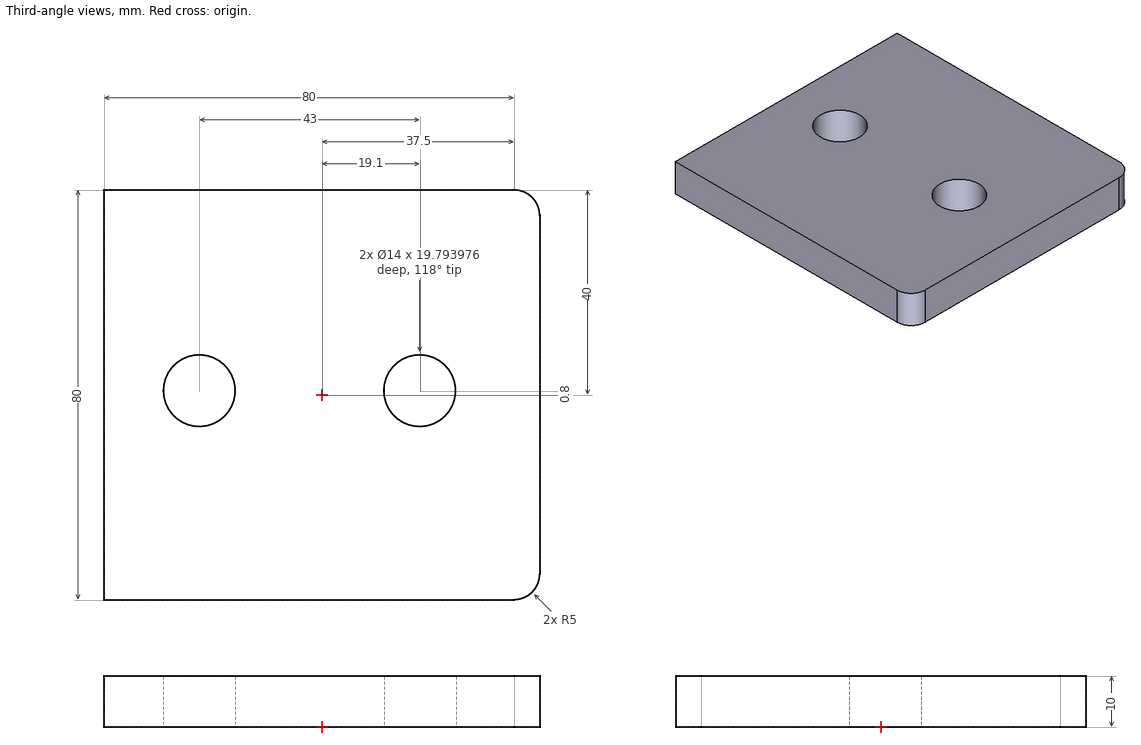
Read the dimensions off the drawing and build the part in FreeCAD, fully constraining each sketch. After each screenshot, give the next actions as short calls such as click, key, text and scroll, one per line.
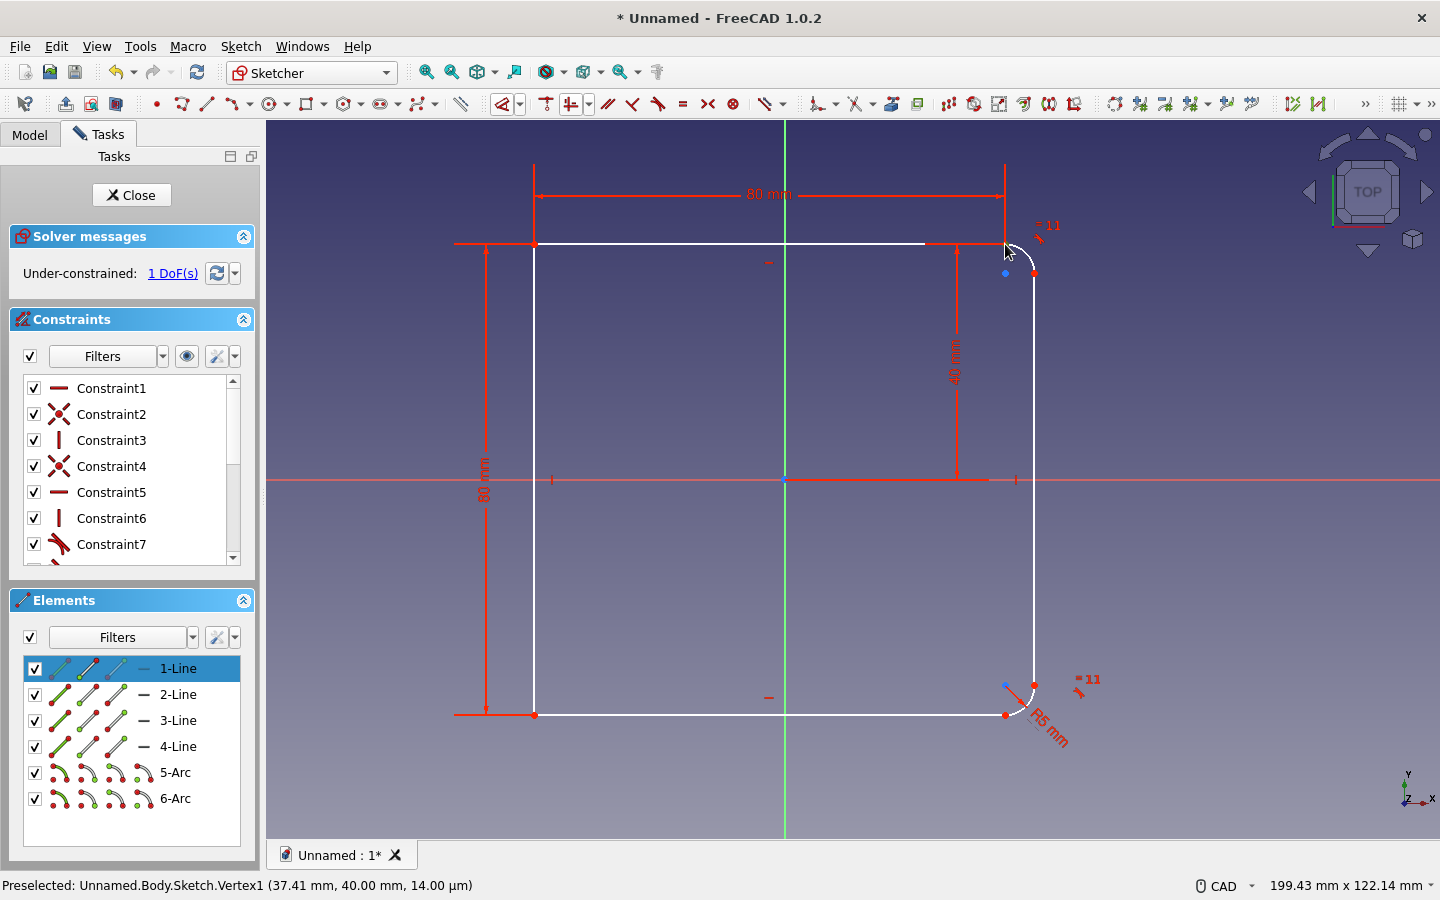
click(520, 104)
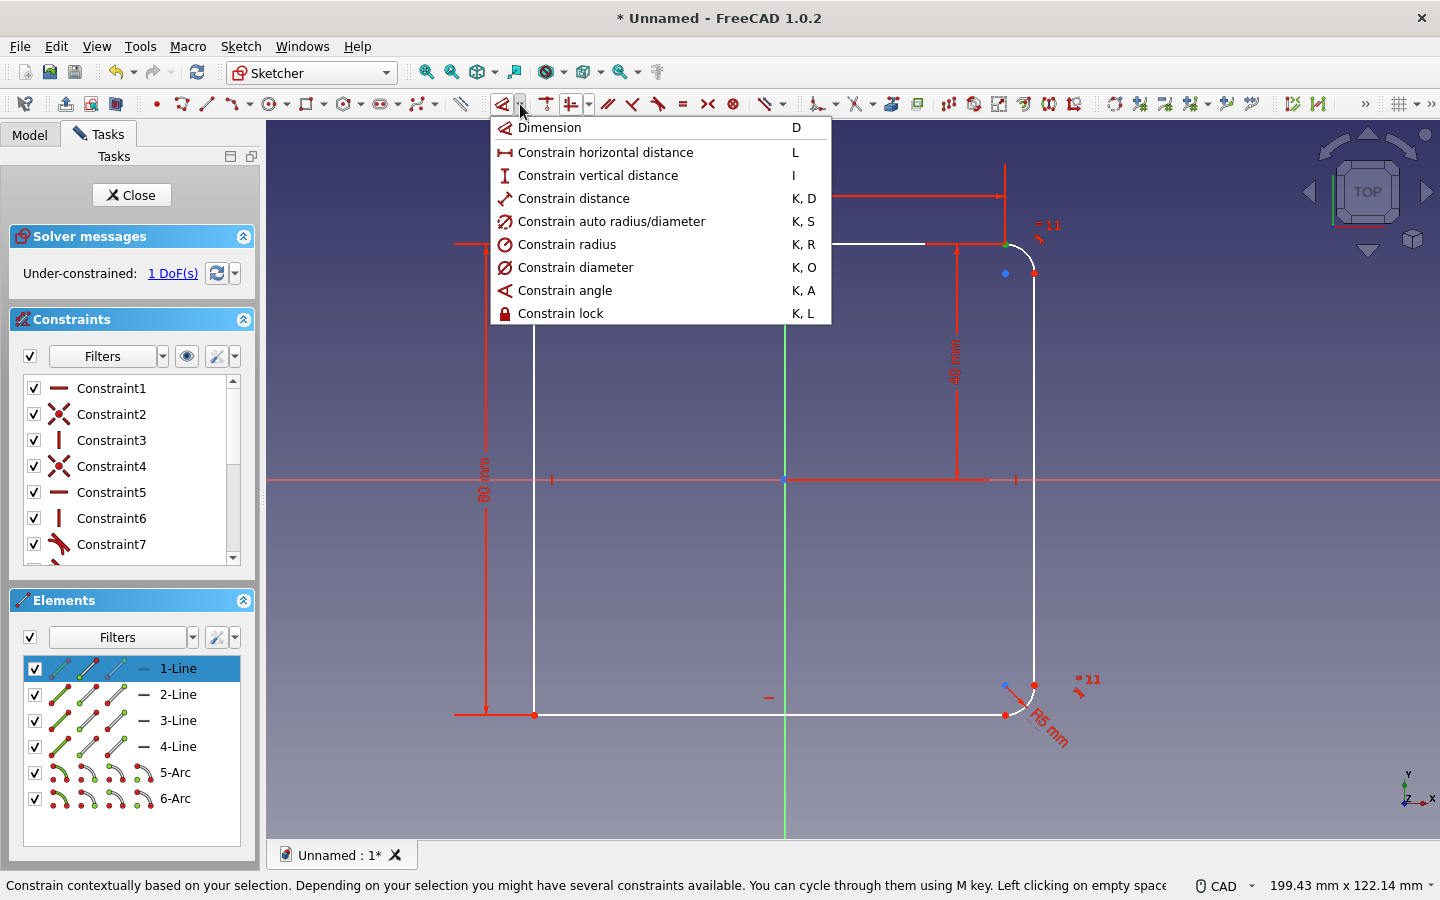
click(661, 152)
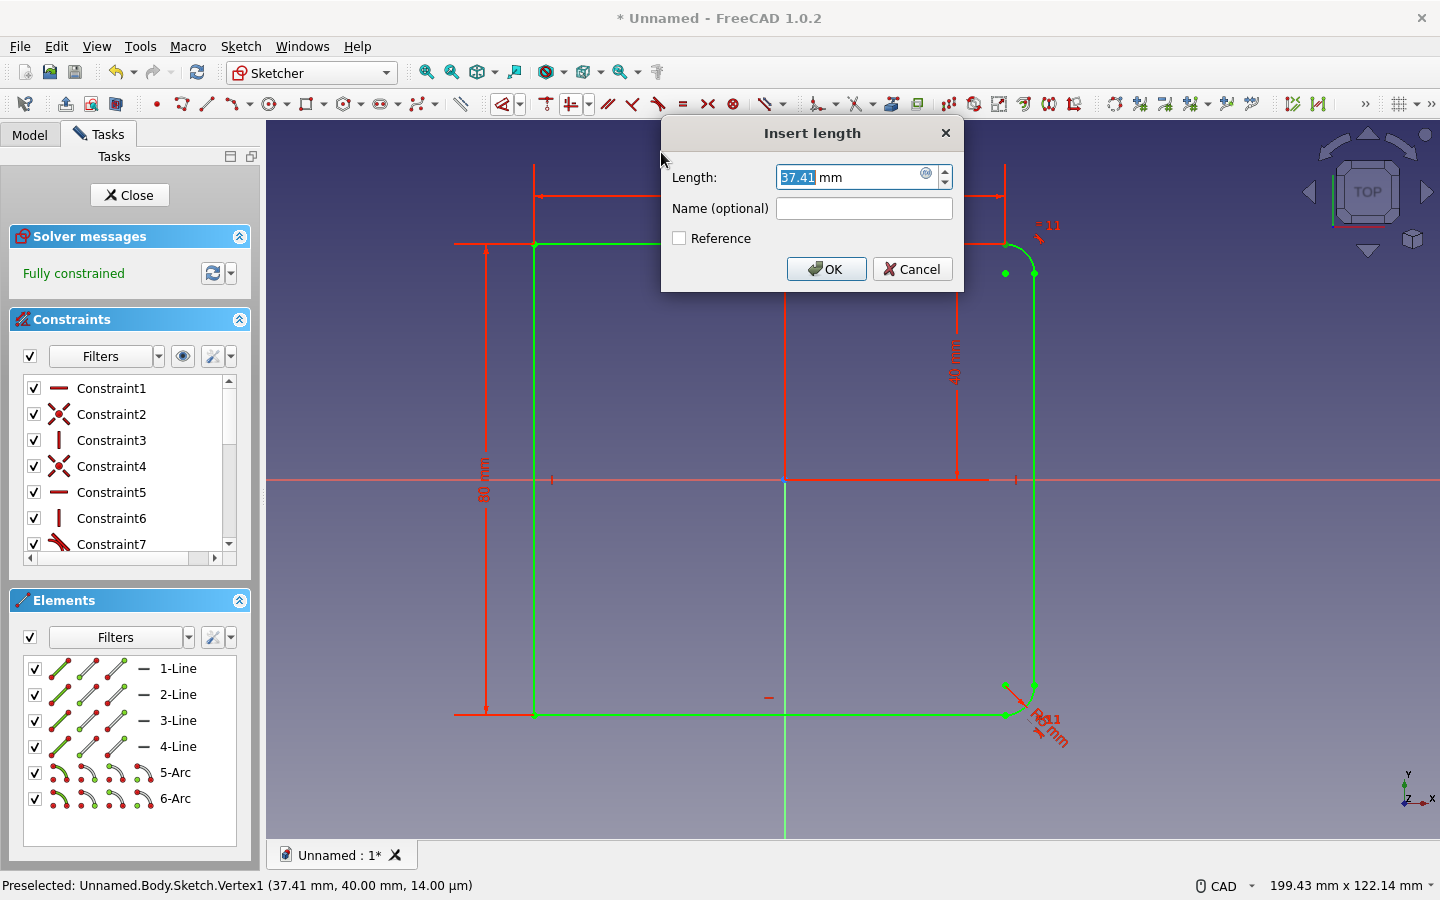
text(37.5)
key(Return)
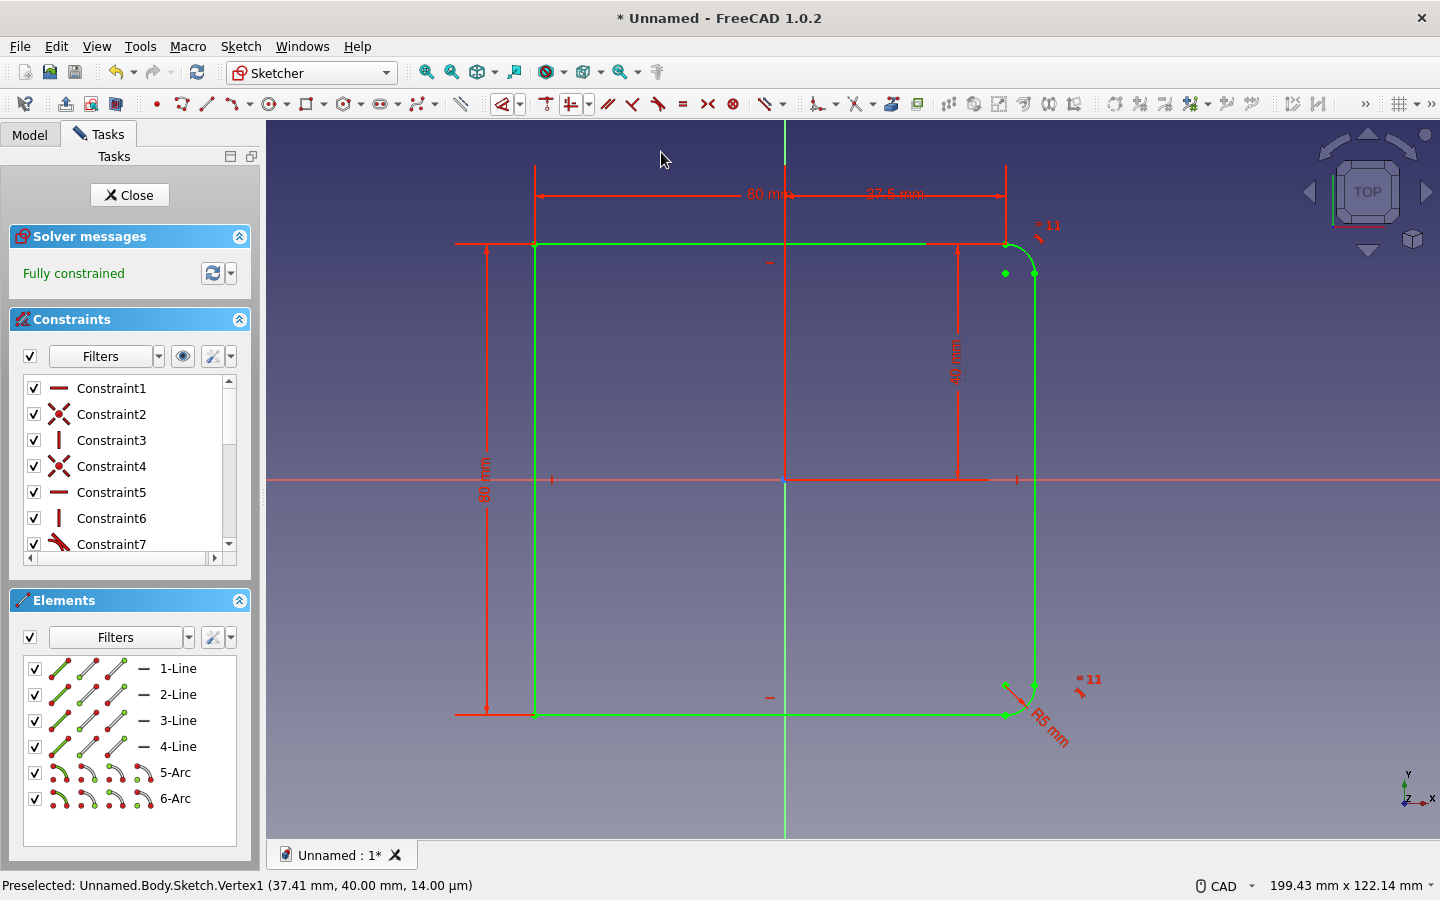
click(130, 195)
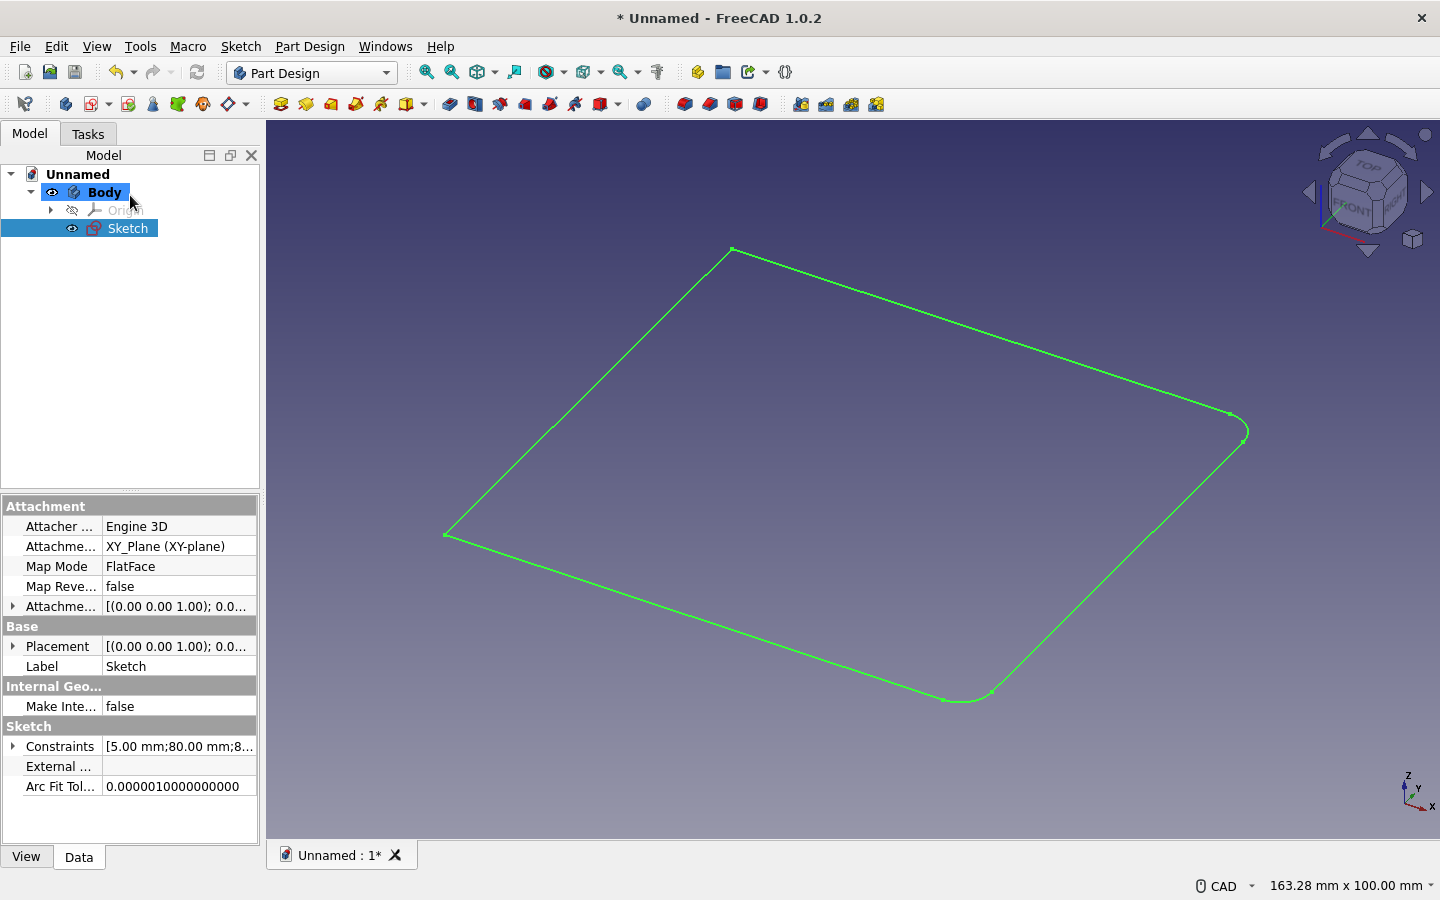
click(281, 104)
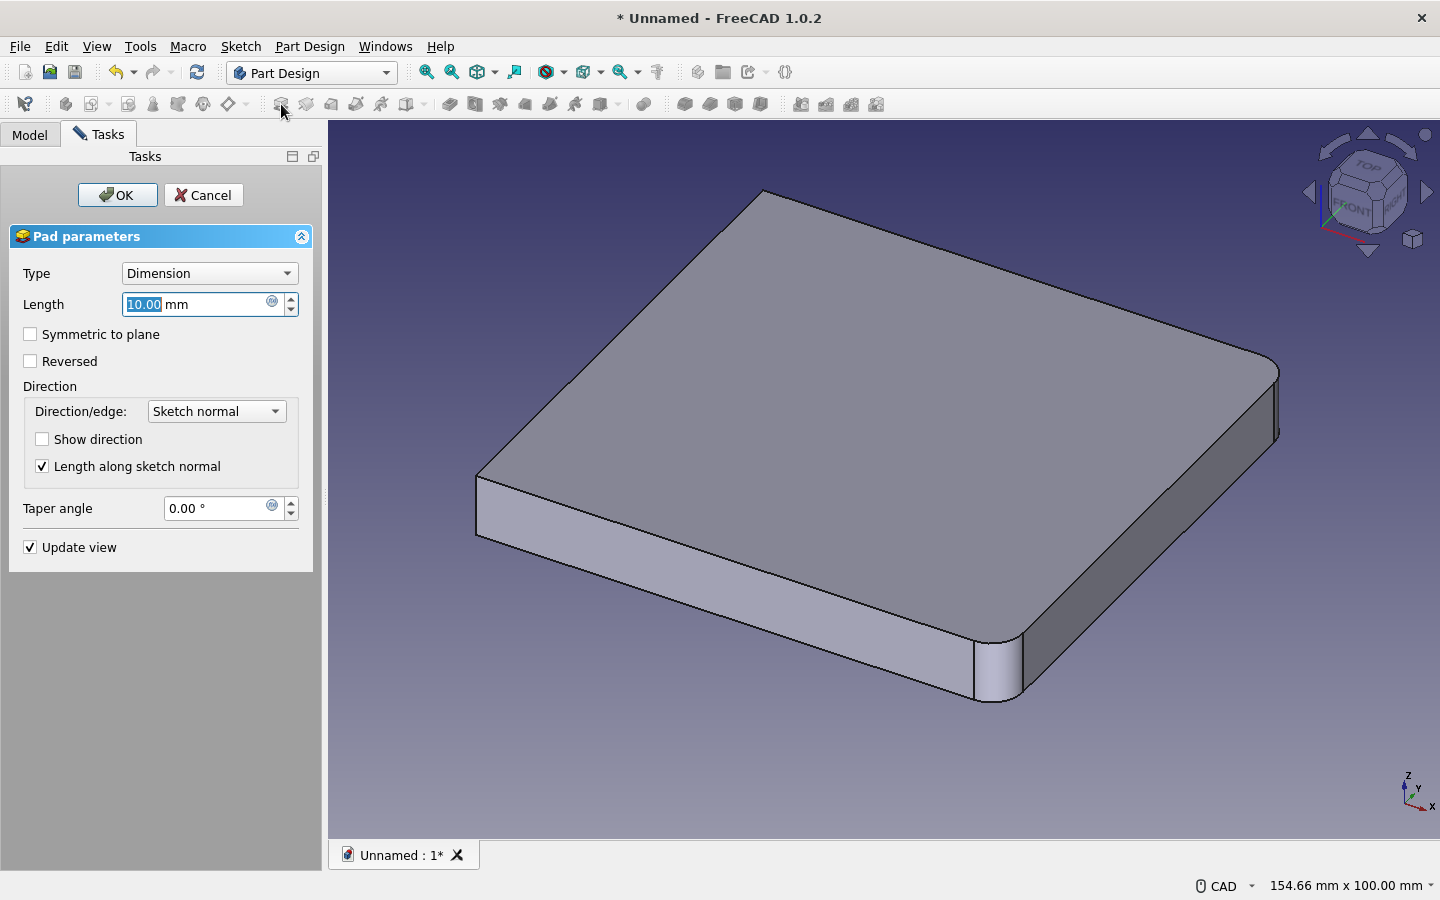
text(10)
key(Tab)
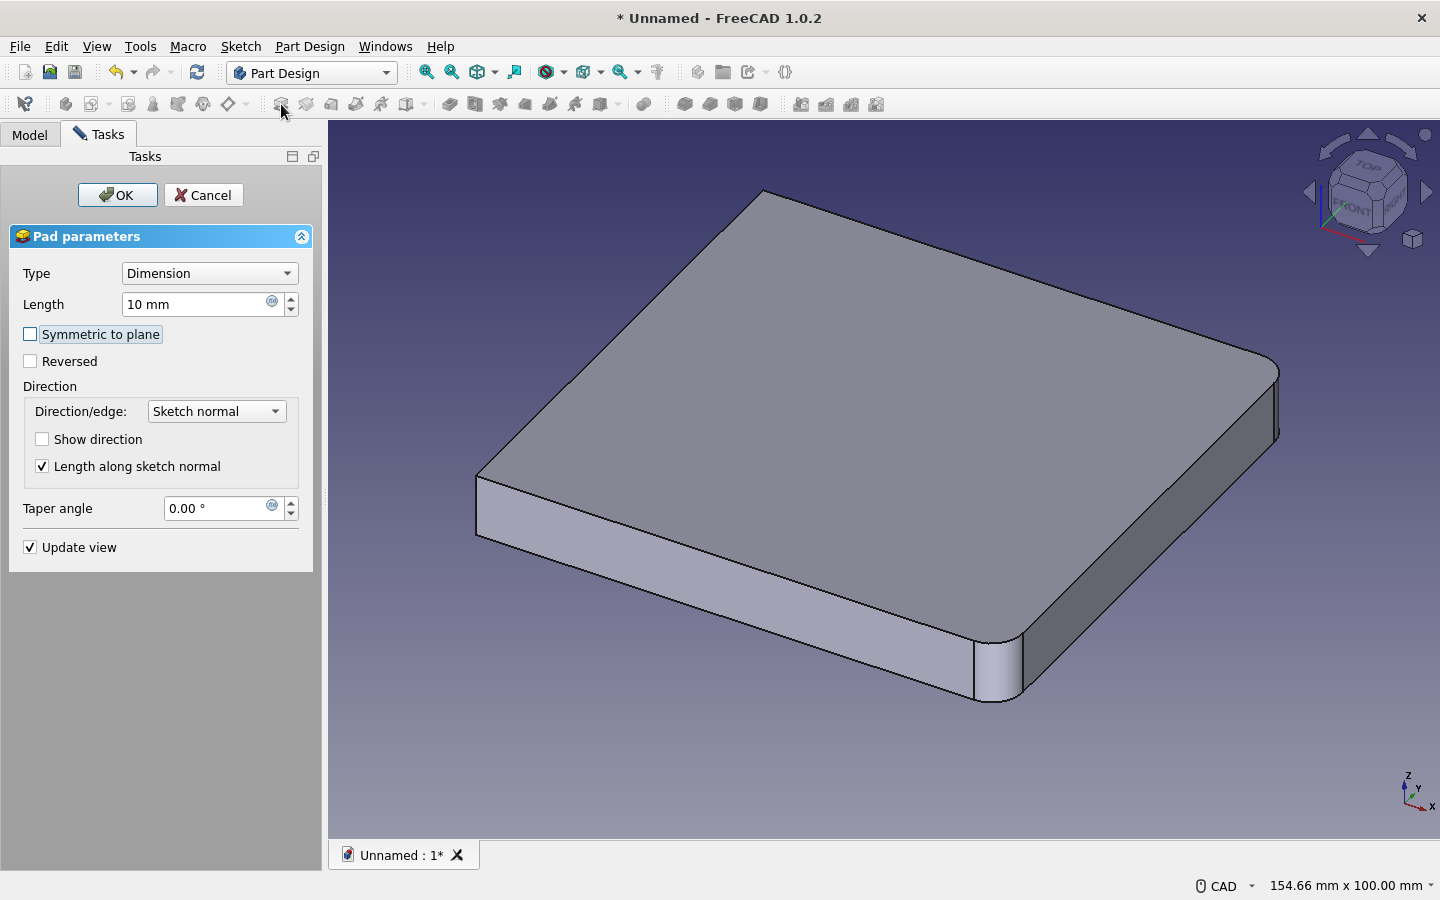
click(118, 195)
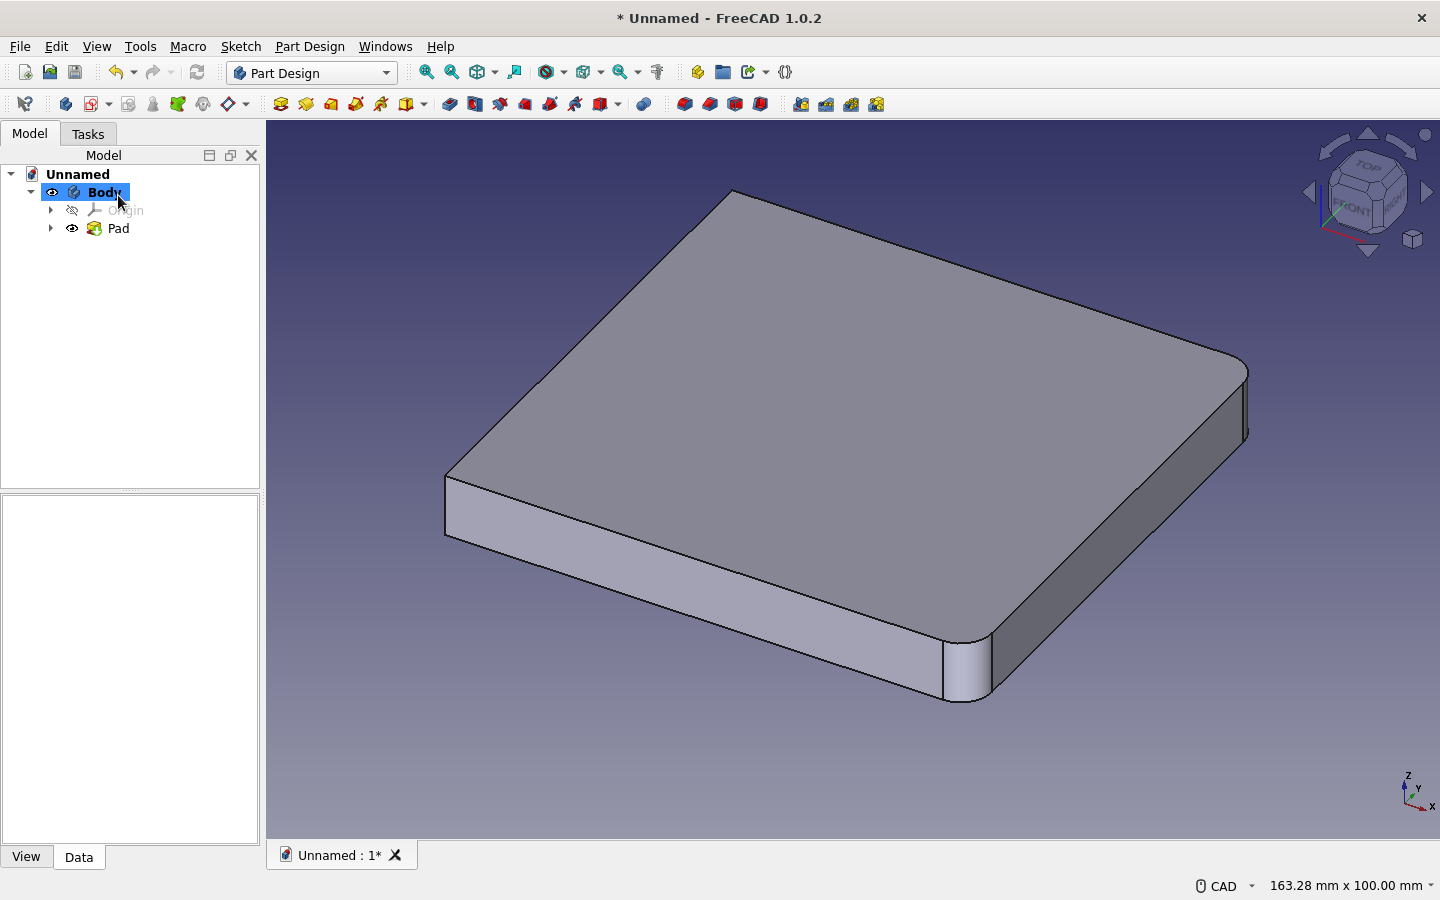
click(853, 420)